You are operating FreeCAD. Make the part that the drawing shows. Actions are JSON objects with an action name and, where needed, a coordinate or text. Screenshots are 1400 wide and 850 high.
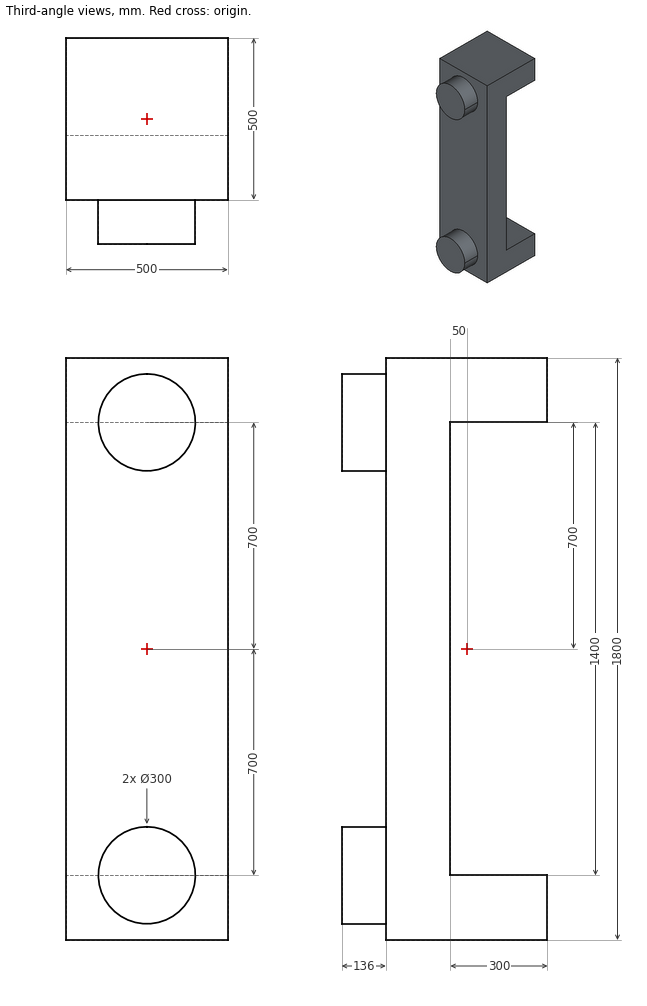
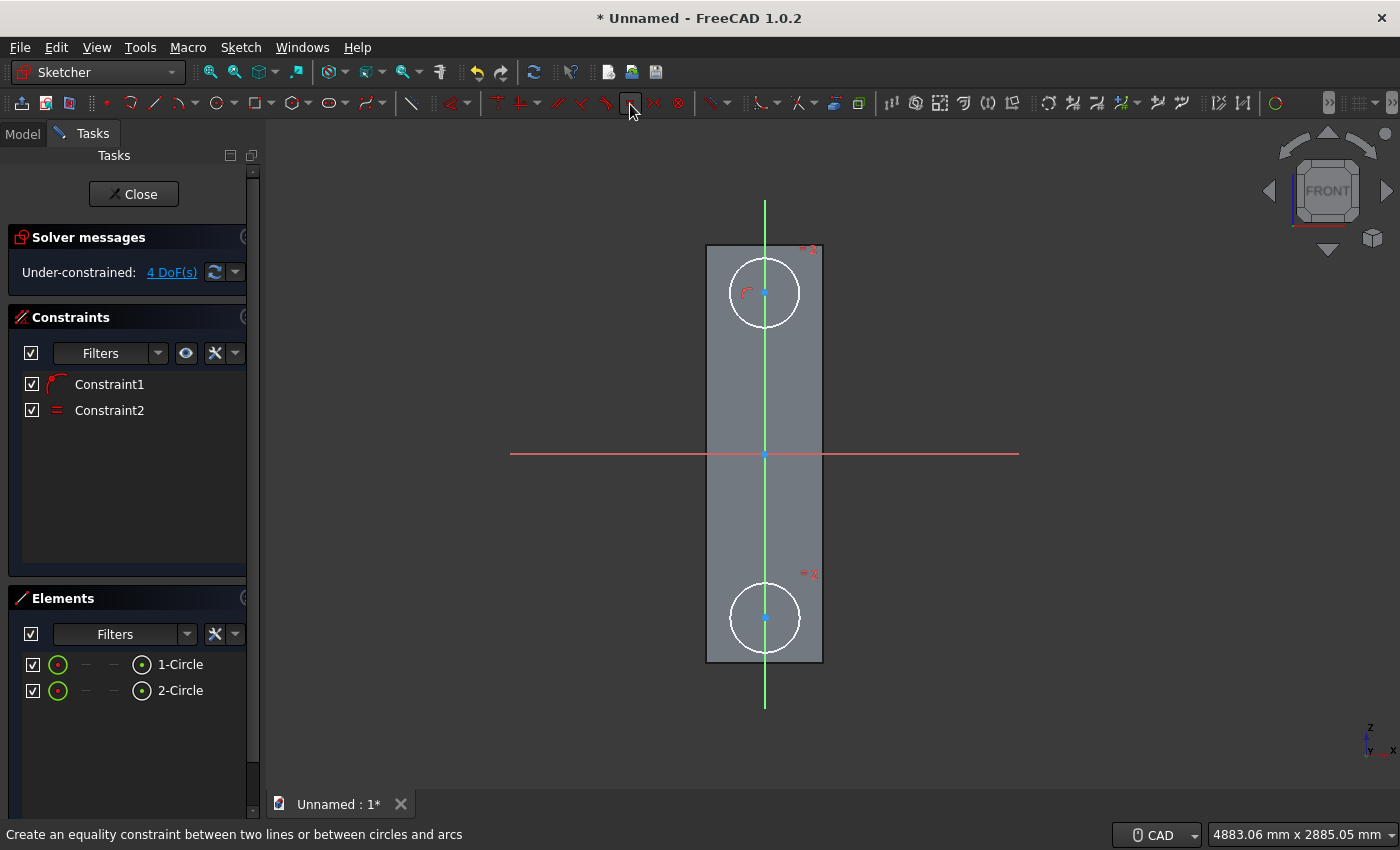
{"action": "left_click", "coordinate": [765, 618]}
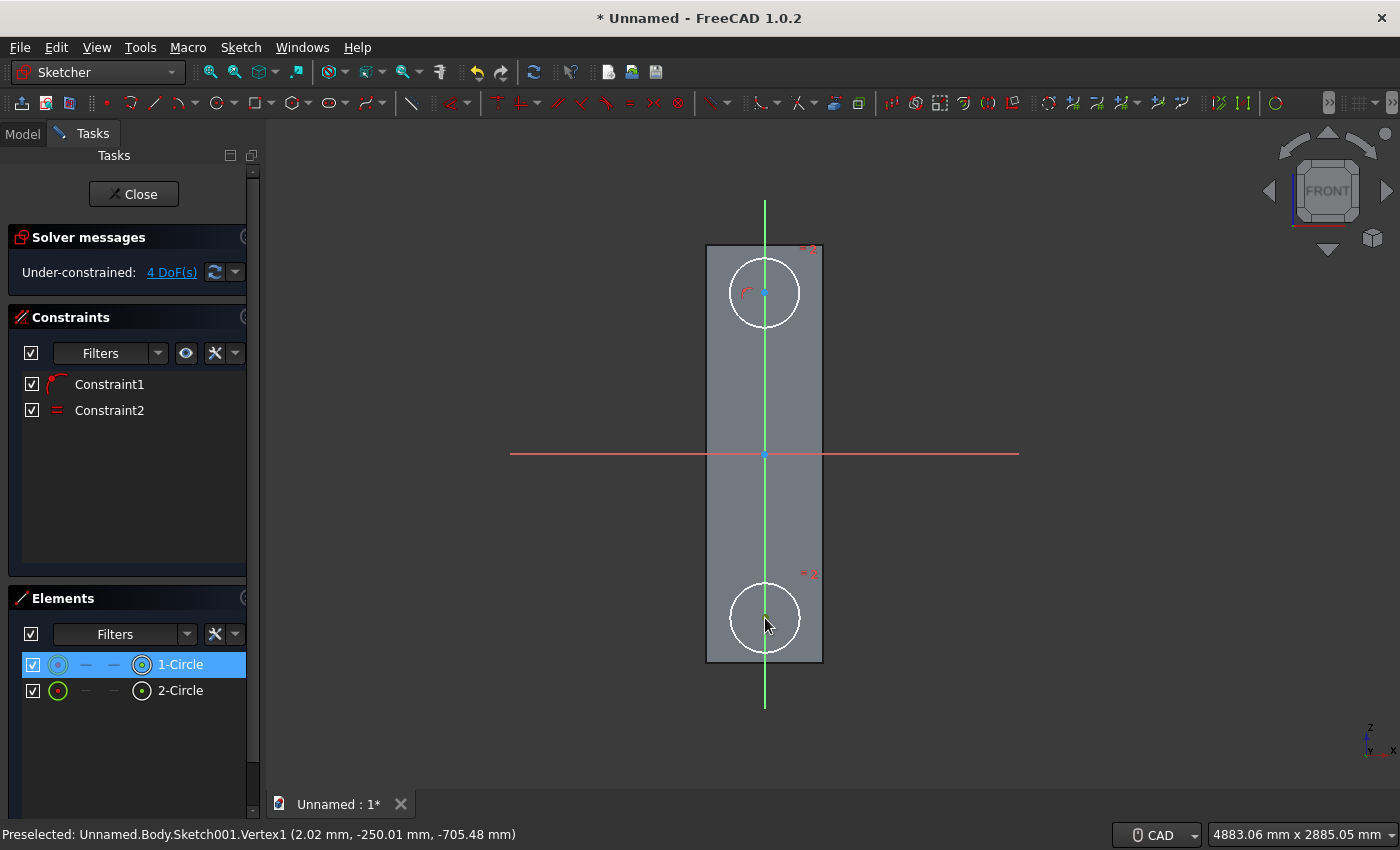
{"action": "left_click", "coordinate": [765, 542]}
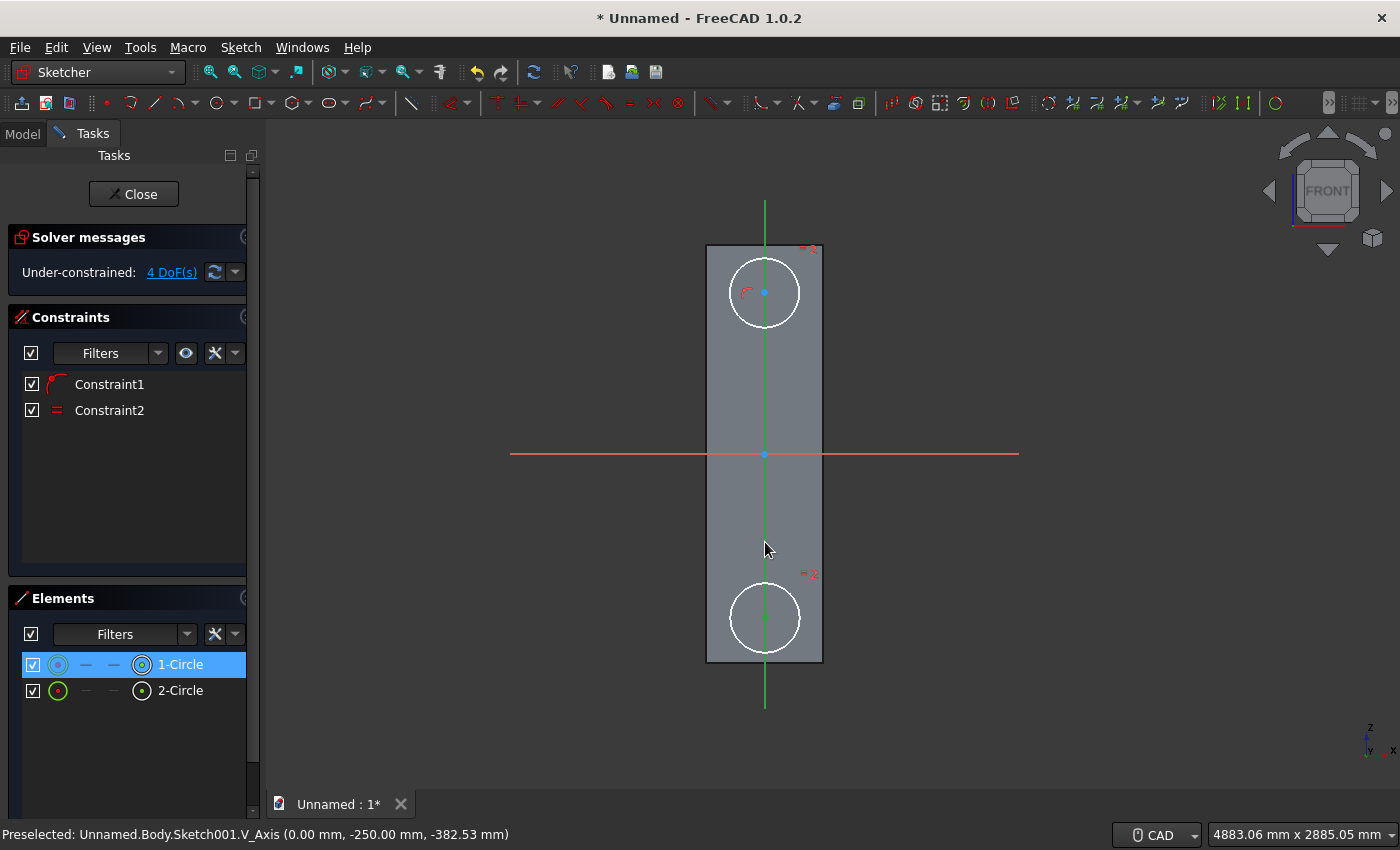
{"action": "left_click", "coordinate": [498, 104]}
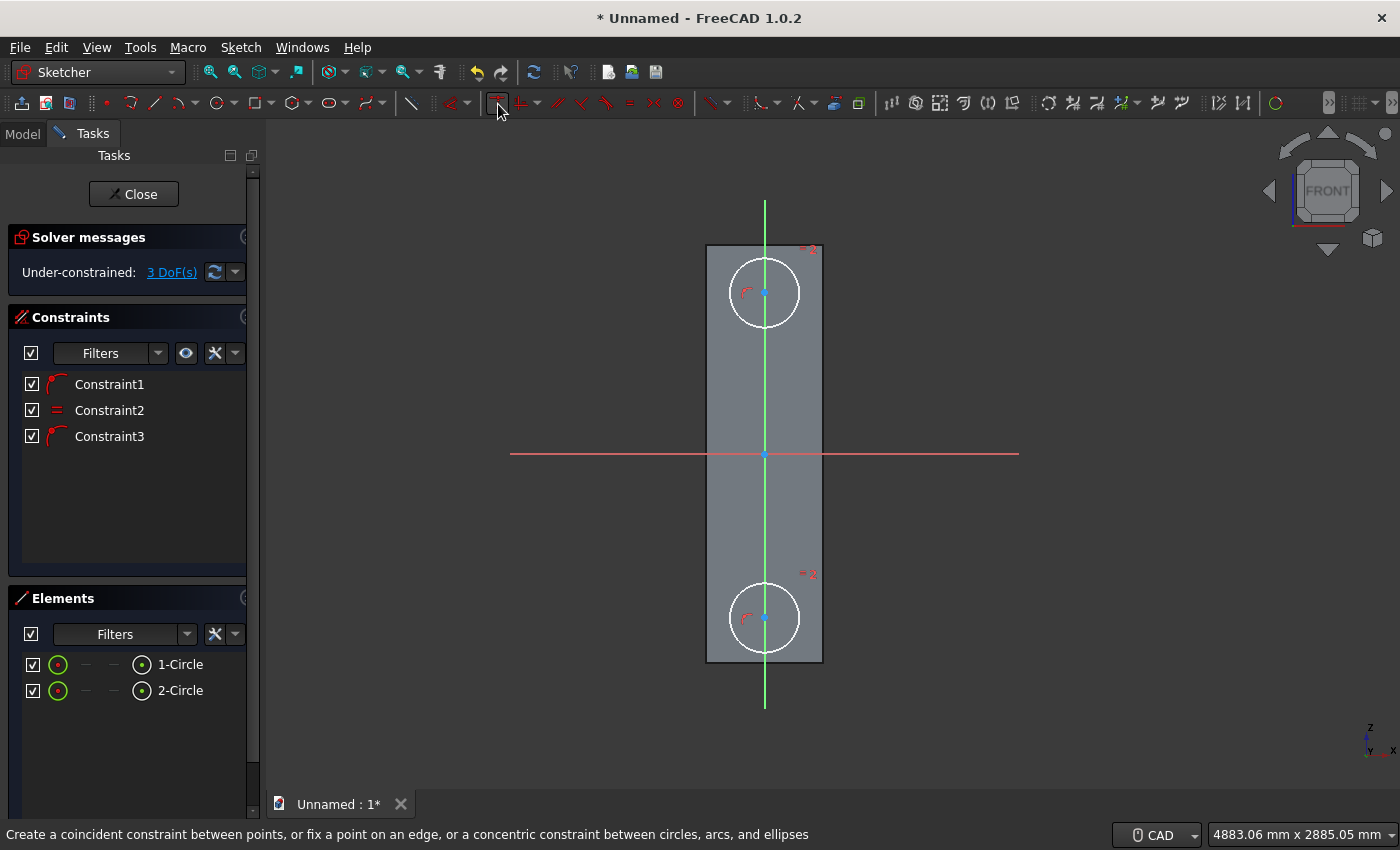
{"action": "left_click", "coordinate": [450, 104]}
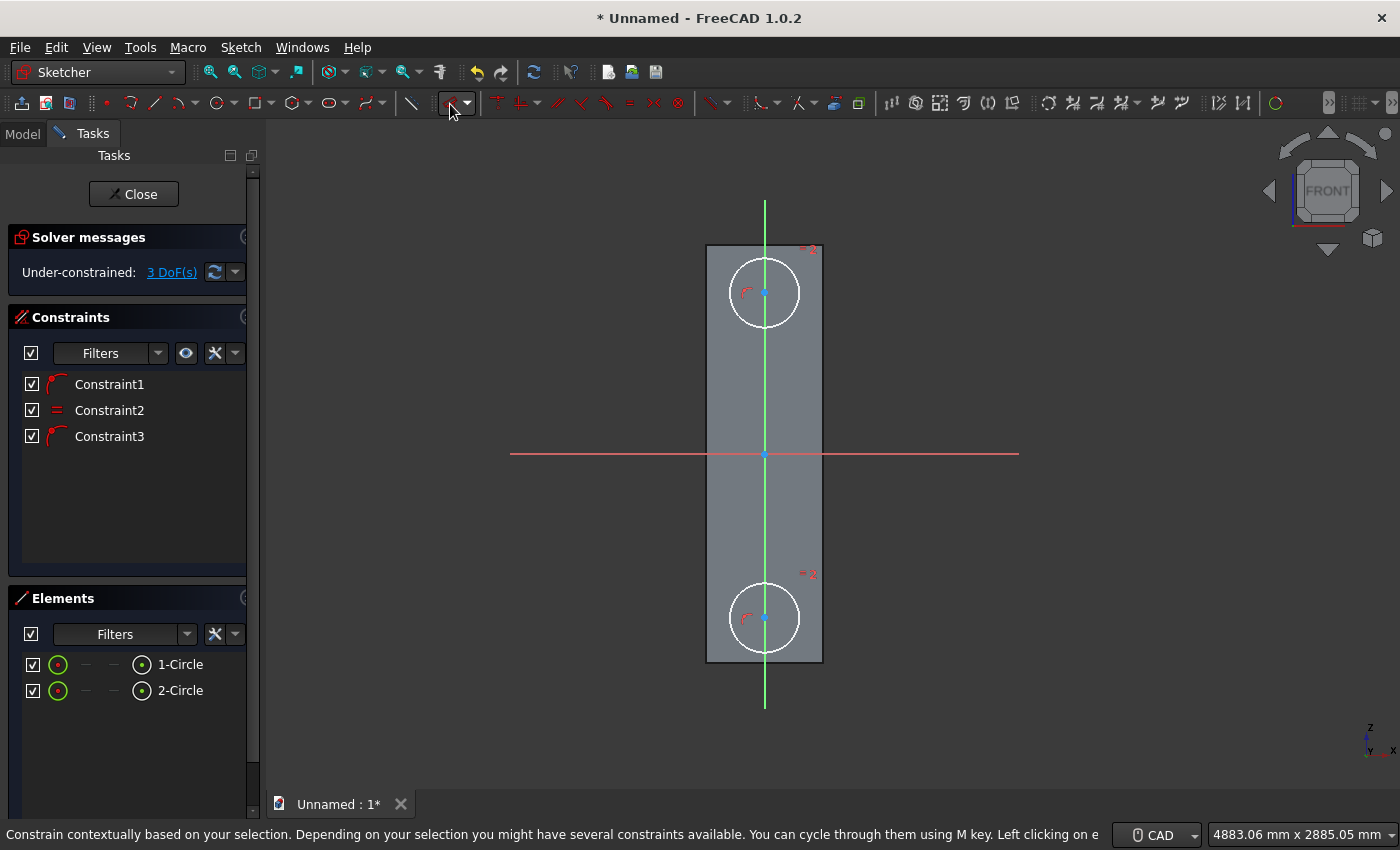
{"action": "left_click", "coordinate": [789, 593]}
{"action": "left_click", "coordinate": [811, 570]}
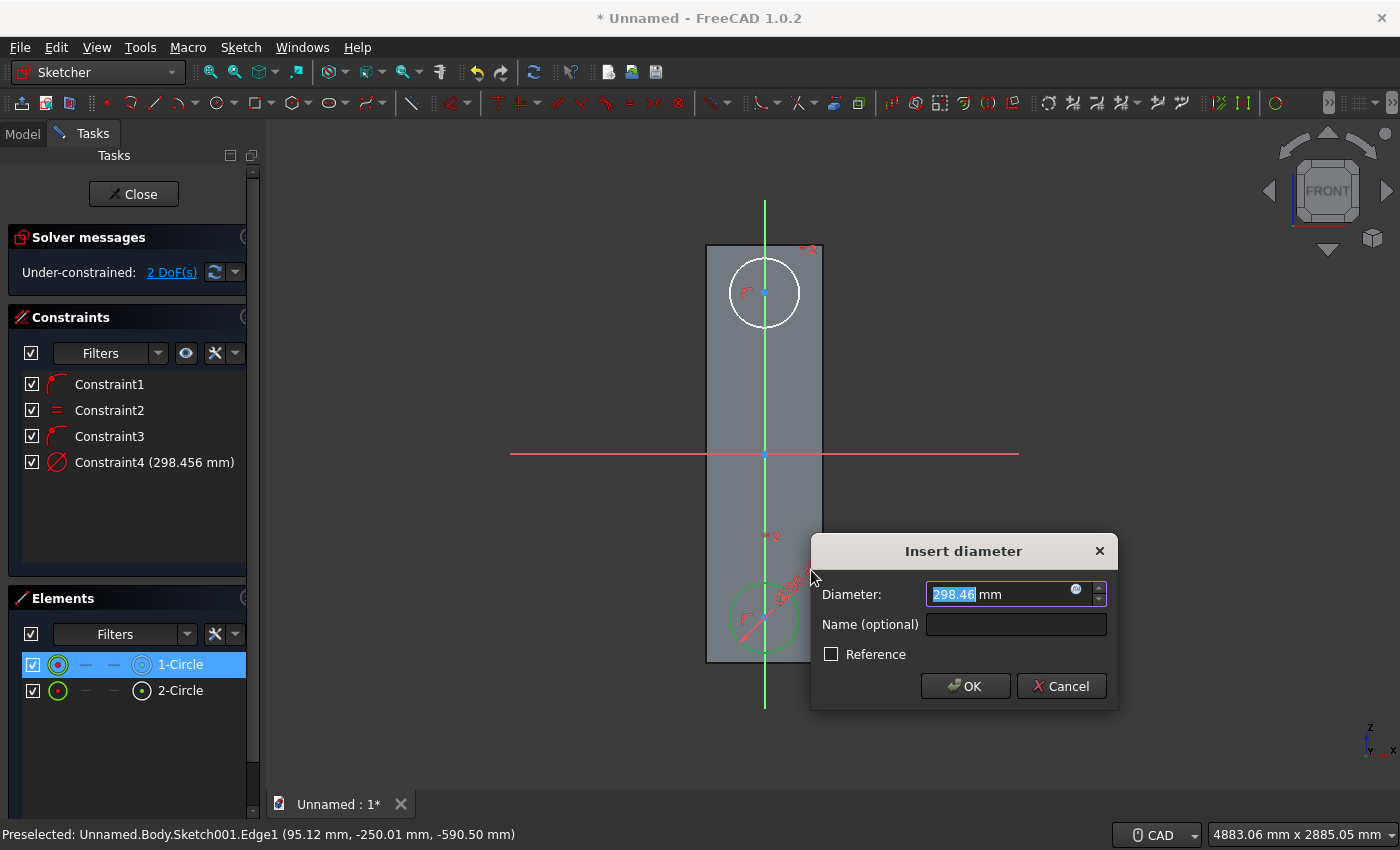
{"action": "type", "text": "300"}
{"action": "key", "text": "Return"}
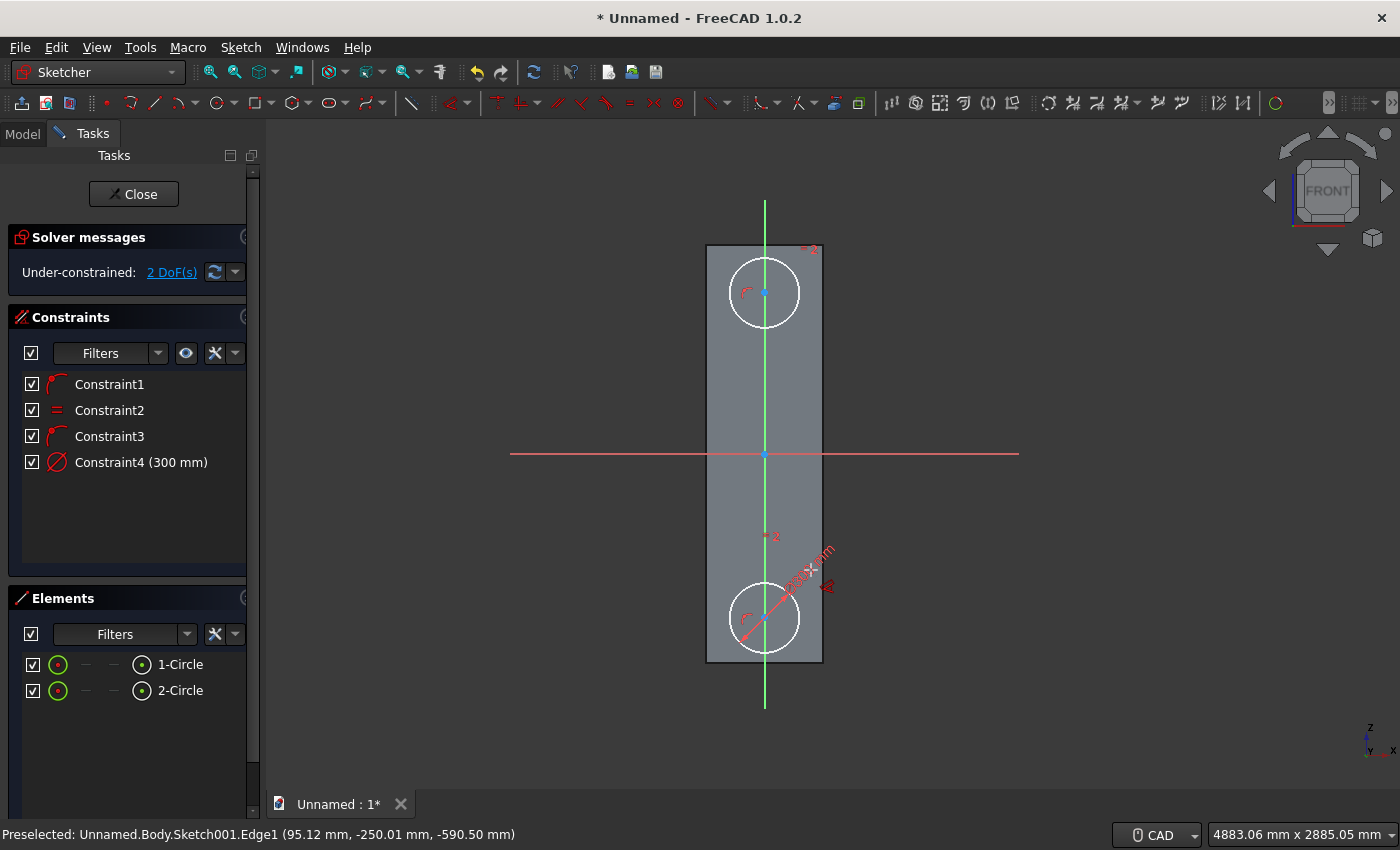
{"action": "left_click", "coordinate": [765, 618]}
{"action": "left_click", "coordinate": [799, 536]}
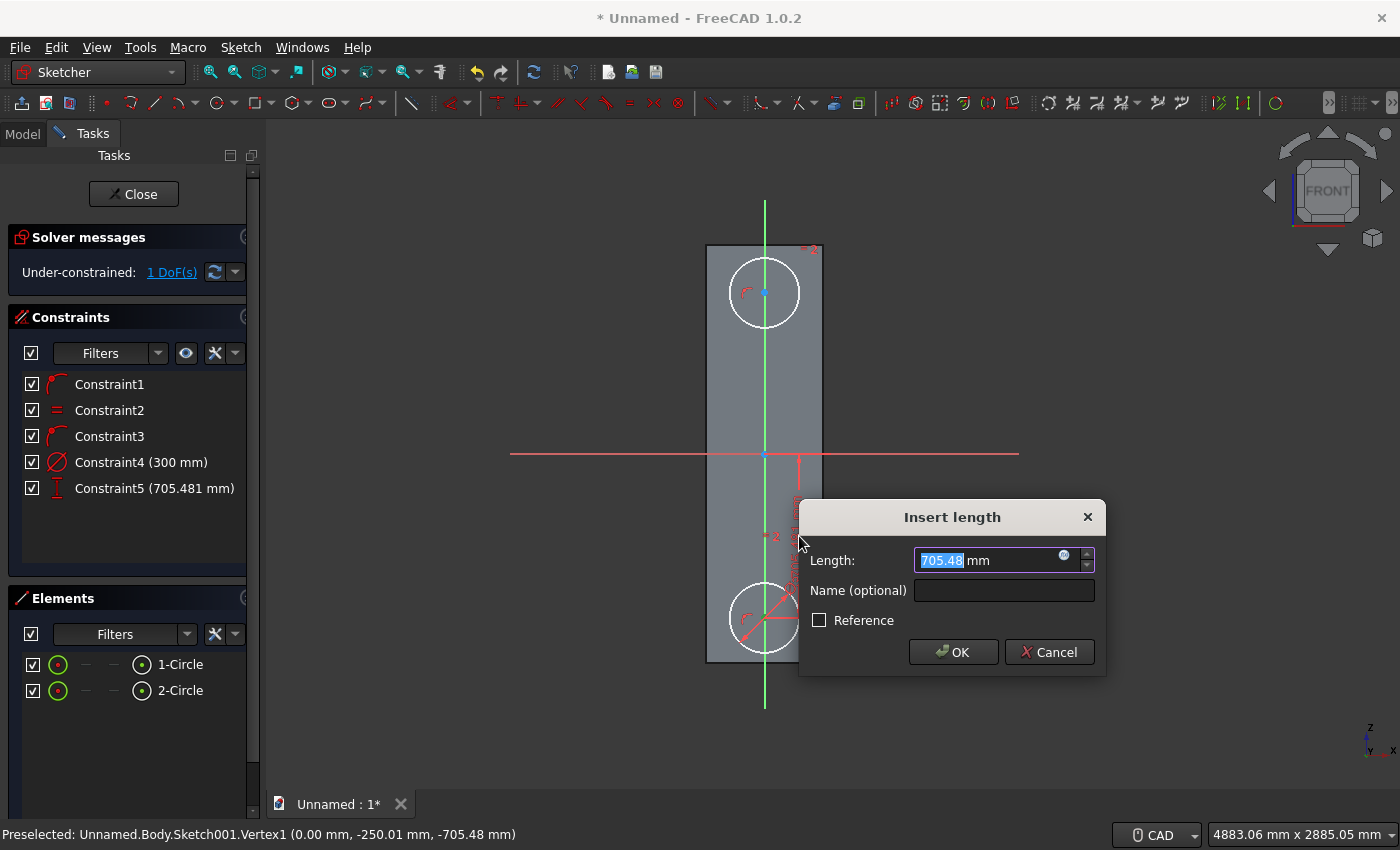
{"action": "type", "text": "700"}
{"action": "key", "text": "Return"}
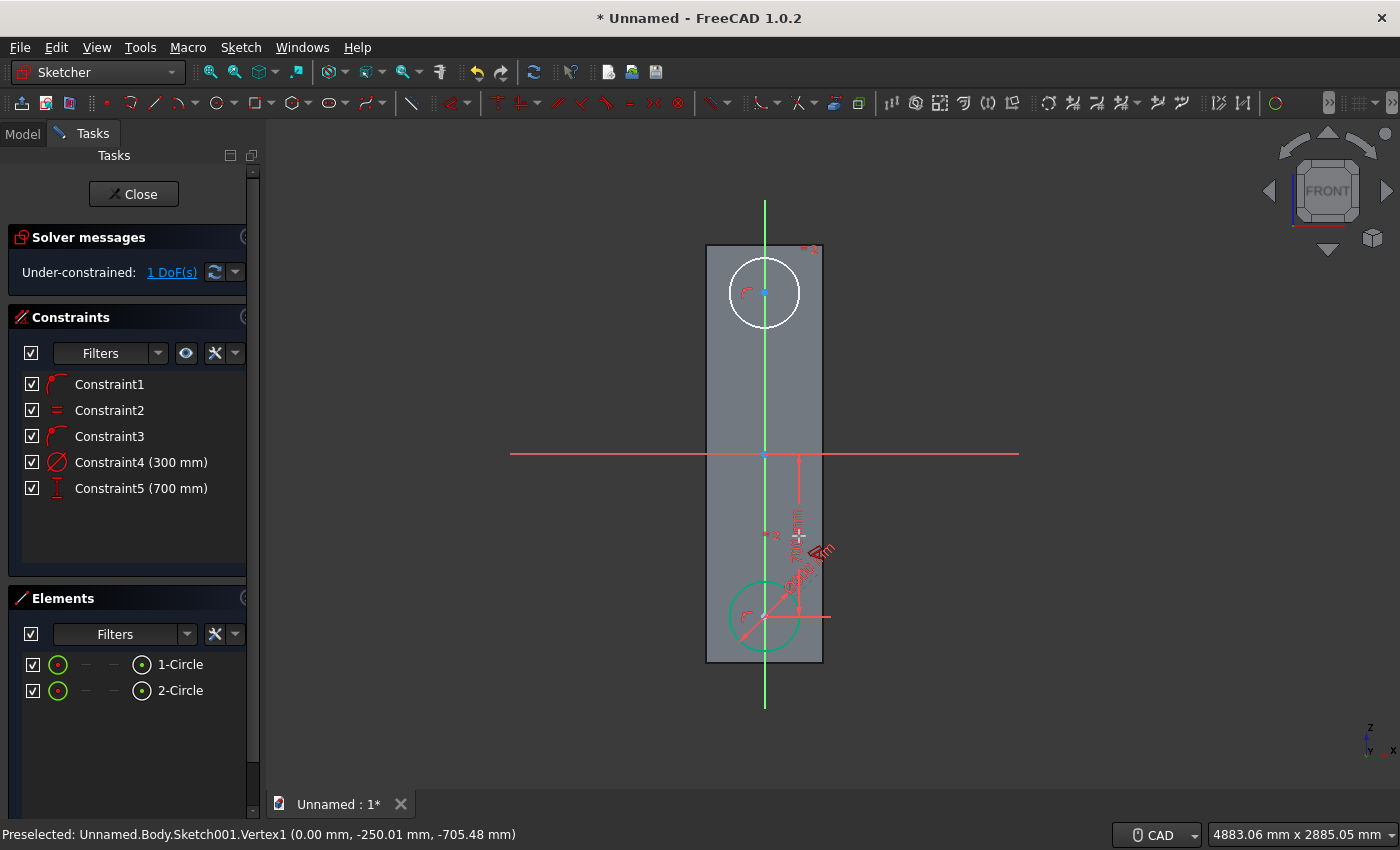
{"action": "left_click", "coordinate": [765, 293]}
{"action": "left_click", "coordinate": [799, 374]}